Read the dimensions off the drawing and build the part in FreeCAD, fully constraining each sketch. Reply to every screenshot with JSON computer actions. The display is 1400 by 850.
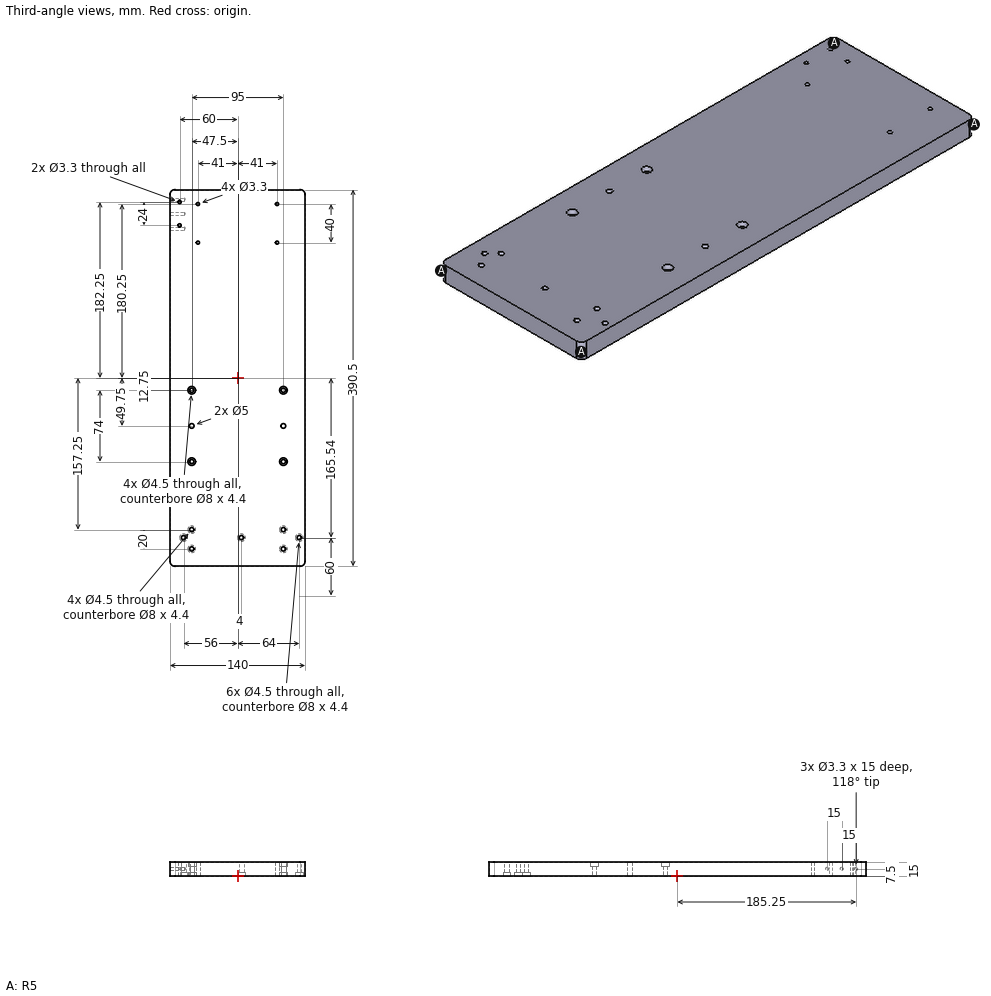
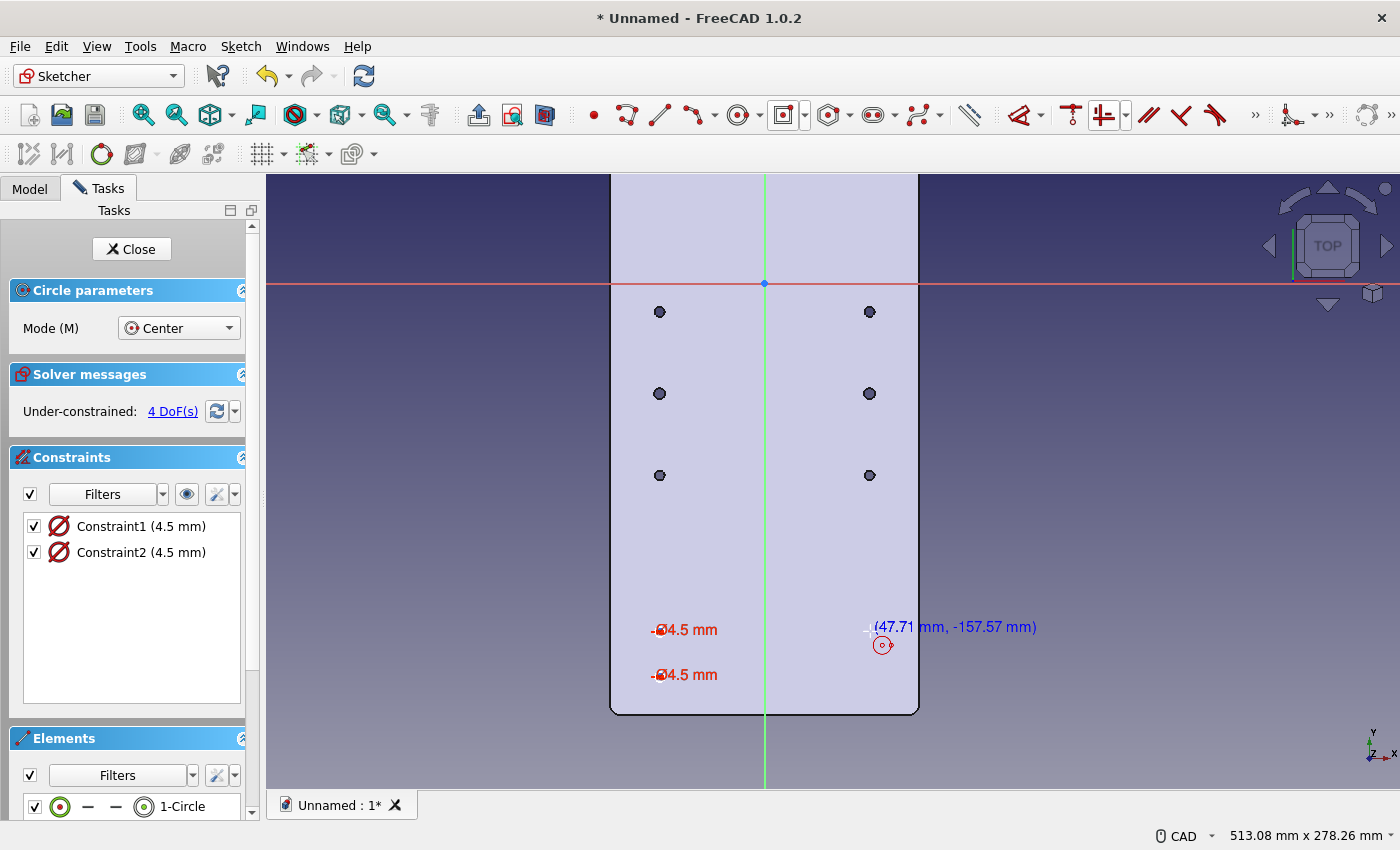
{"action": "left_click", "coordinate": [870, 631]}
{"action": "mouse_move", "coordinate": [873, 628]}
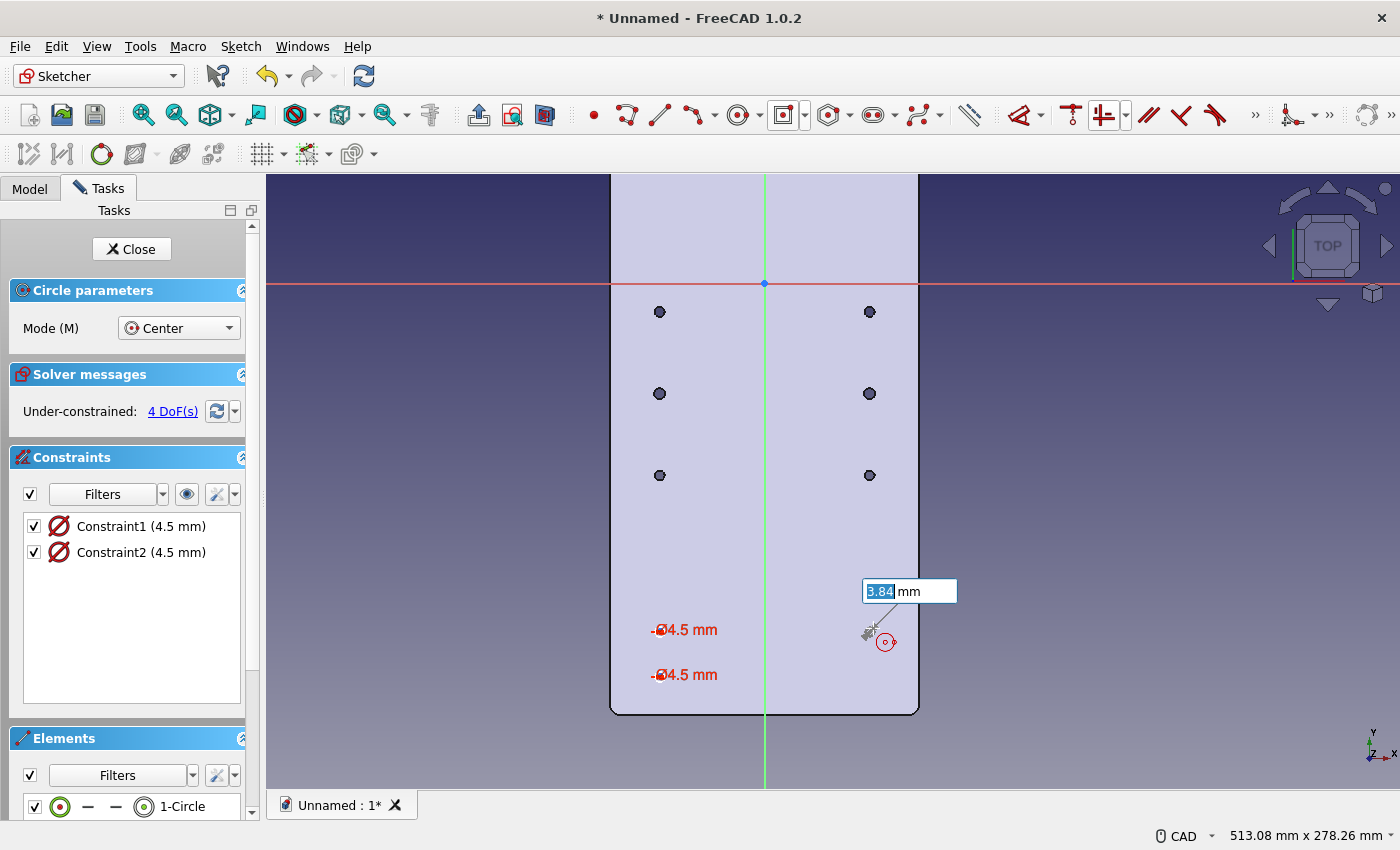
{"action": "type", "text": "4.5"}
{"action": "key", "text": "Return"}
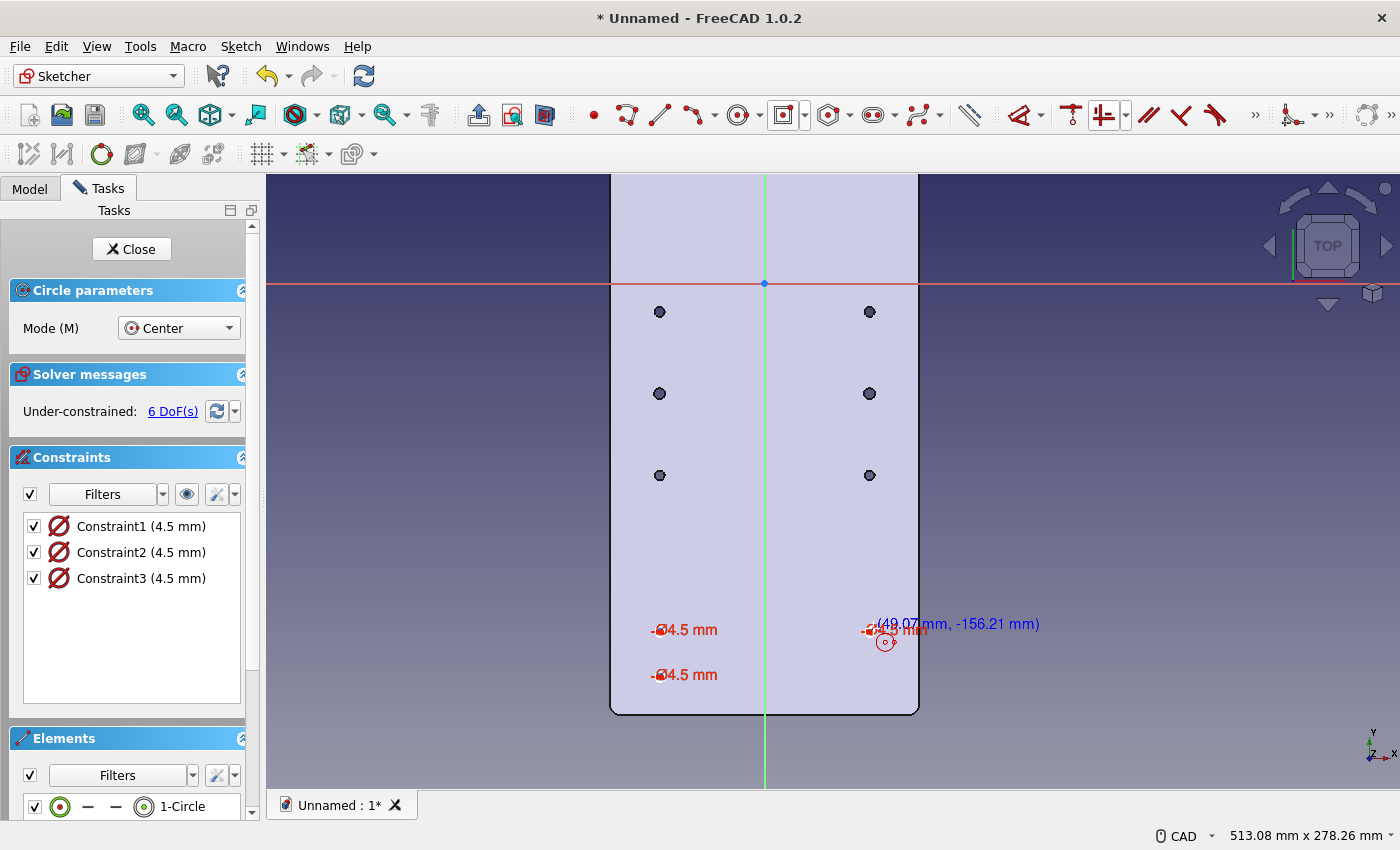
{"action": "scroll", "coordinate": [870, 676], "scroll_direction": "up", "scroll_amount": 8}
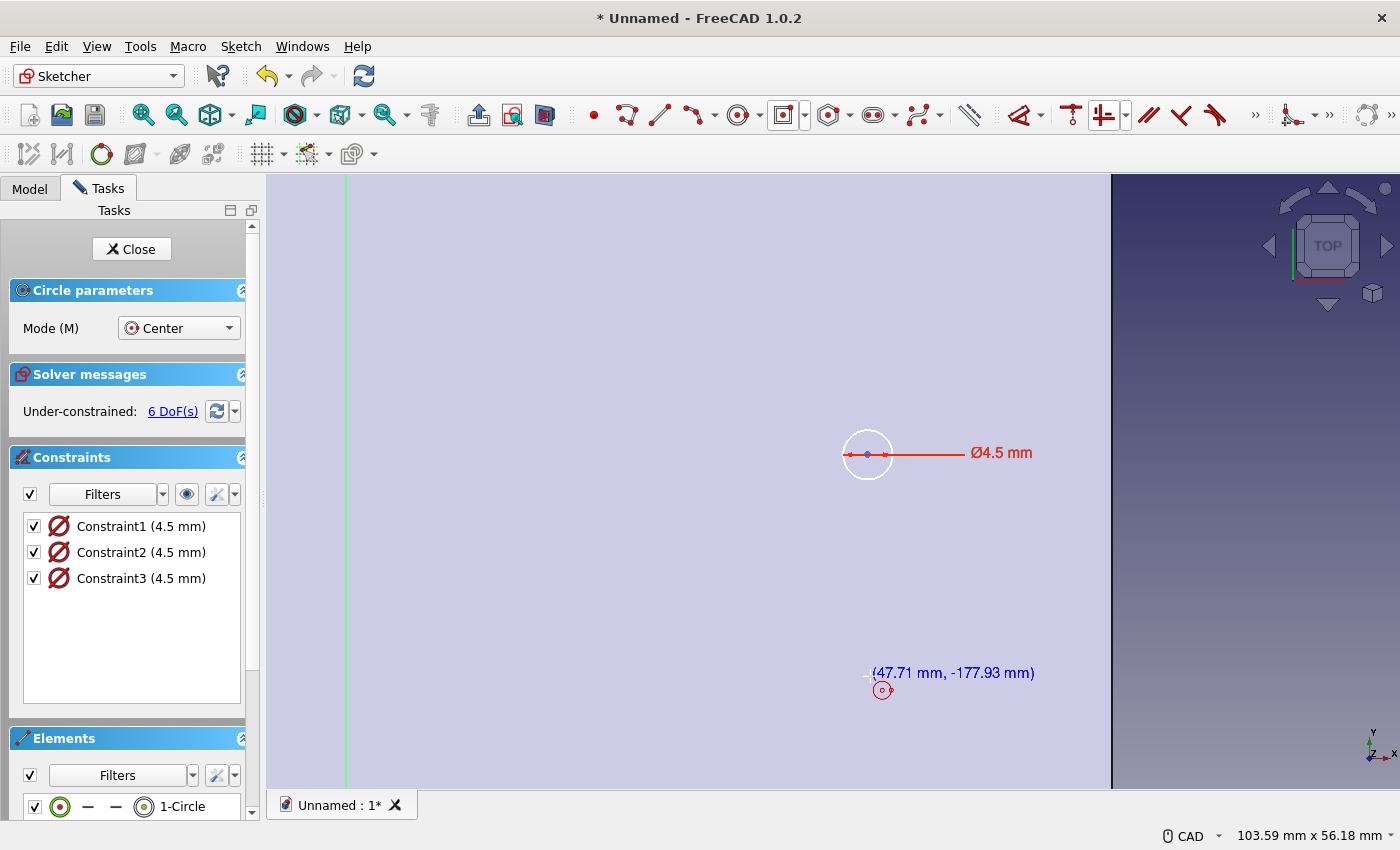
{"action": "scroll", "coordinate": [870, 676], "scroll_direction": "down", "scroll_amount": 8}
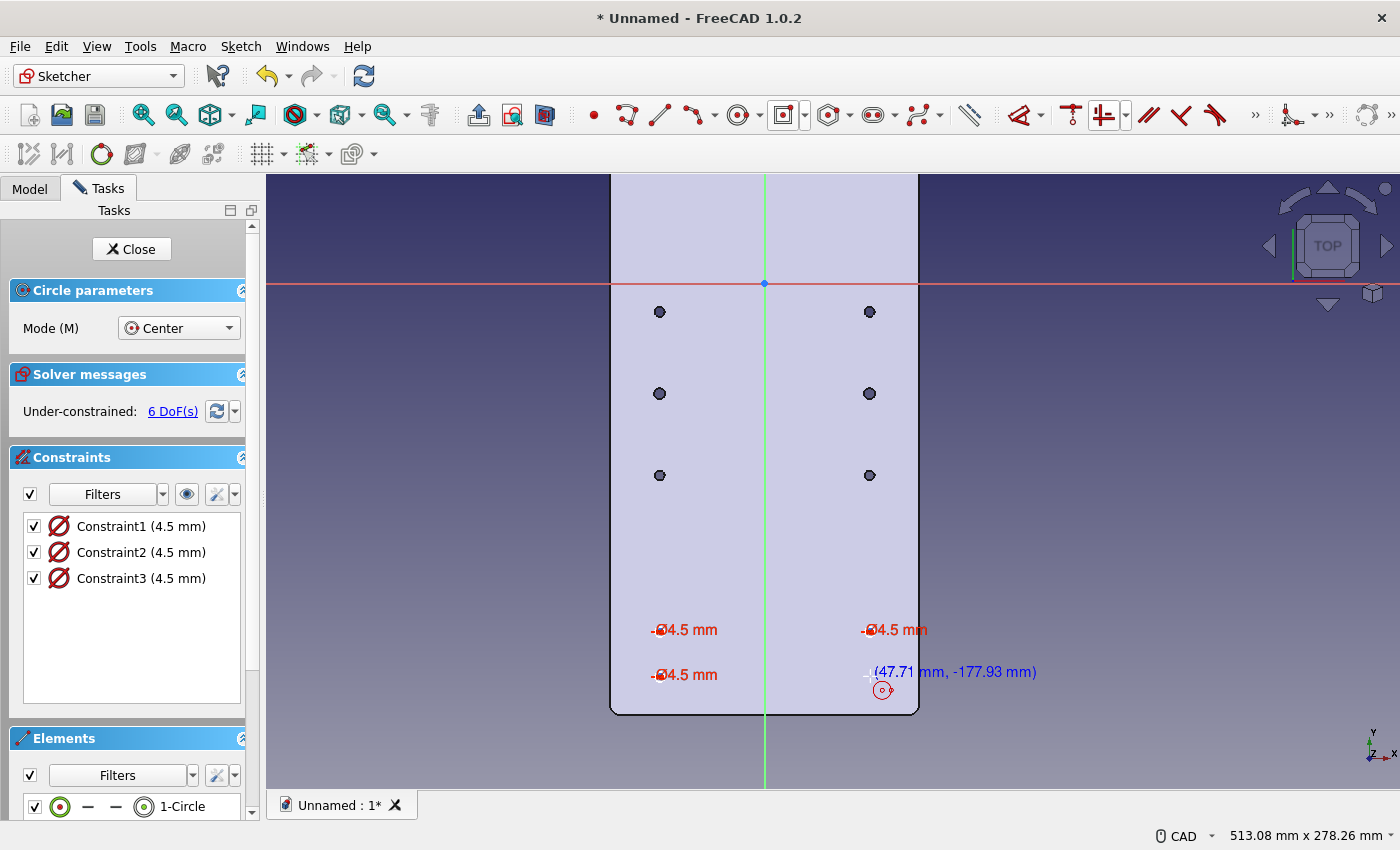
{"action": "left_click", "coordinate": [870, 676]}
{"action": "mouse_move", "coordinate": [873, 672]}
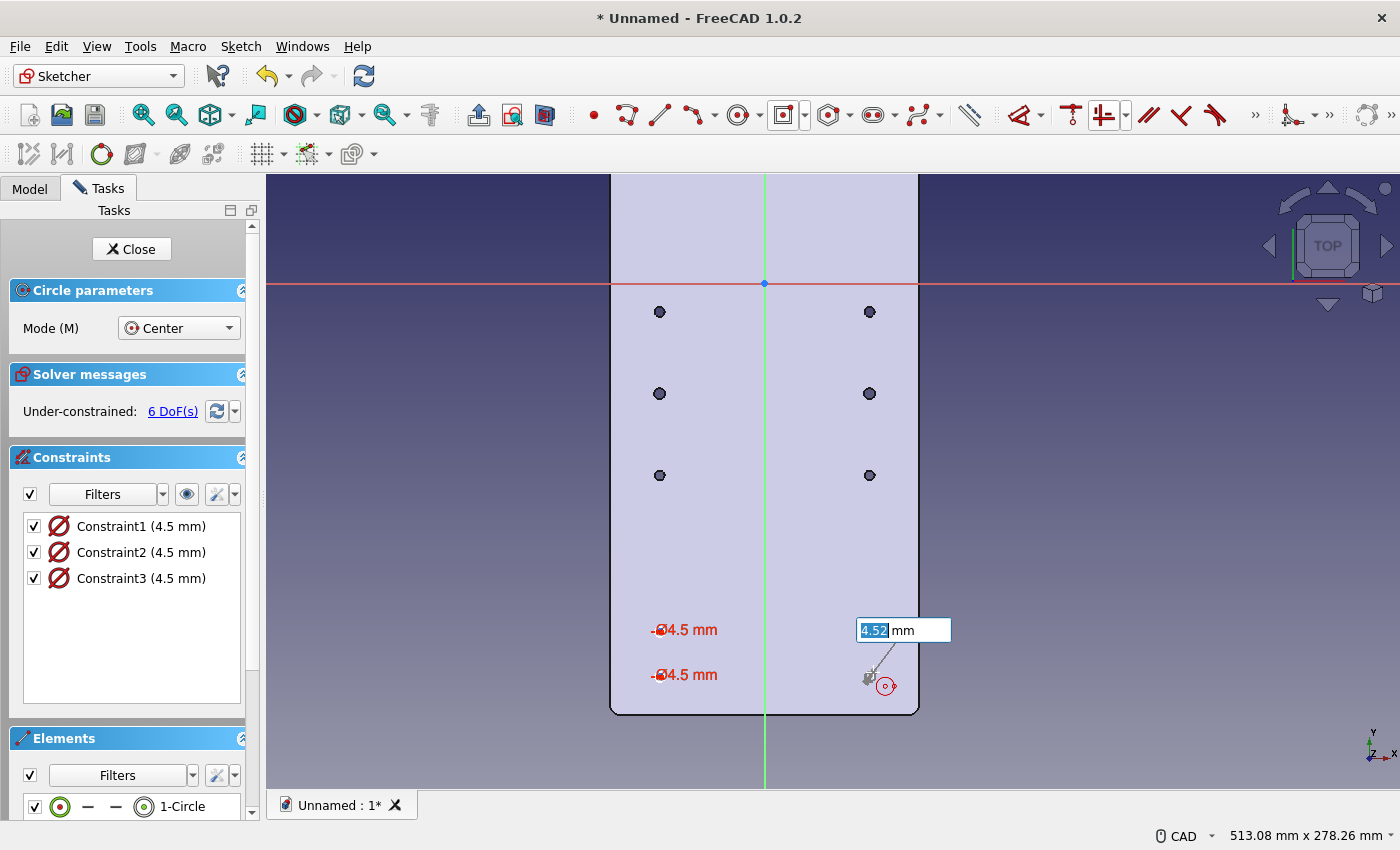
{"action": "type", "text": "4.5"}
{"action": "key", "text": "Return"}
{"action": "key", "text": "Escape"}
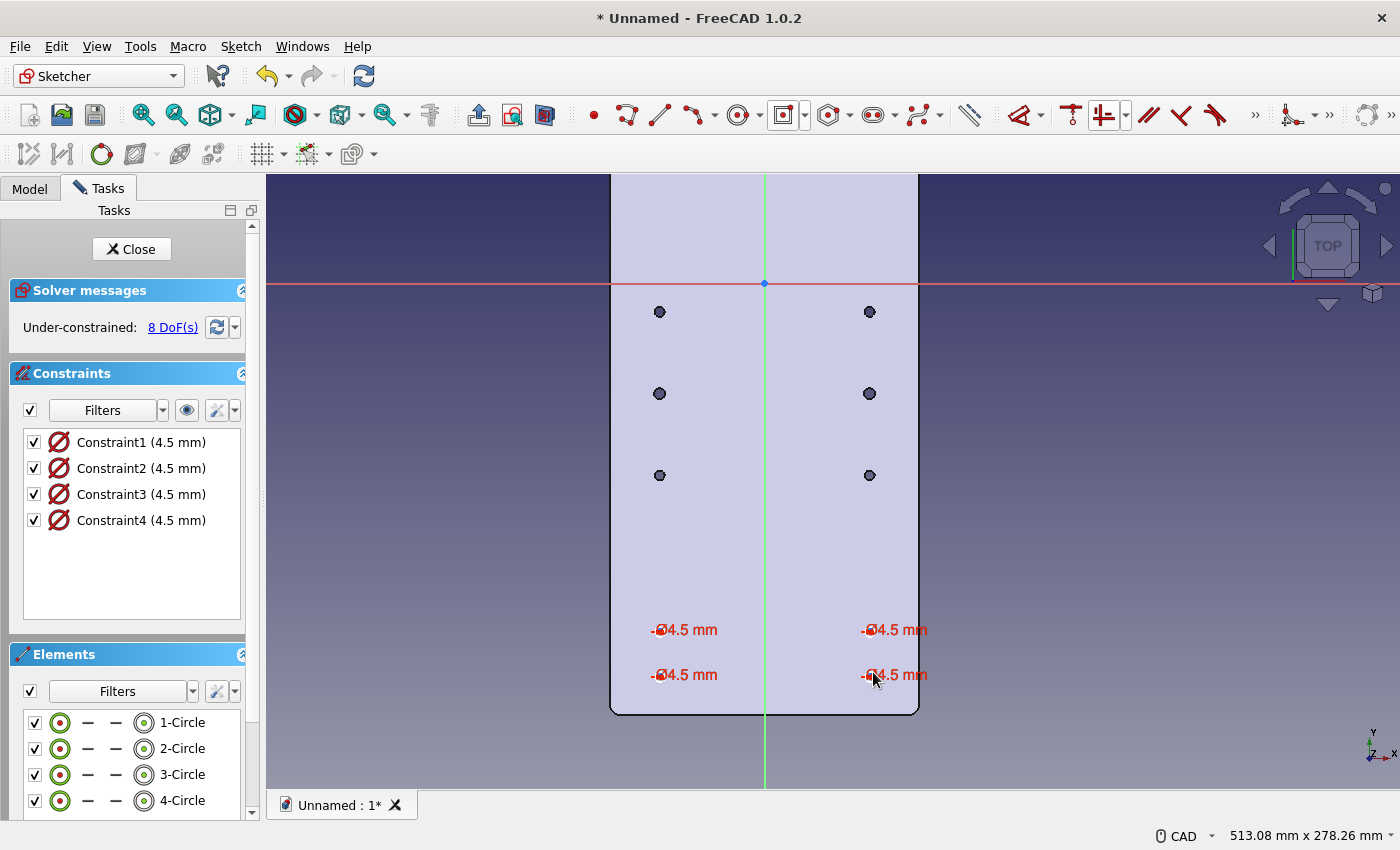
{"action": "left_click", "coordinate": [660, 632]}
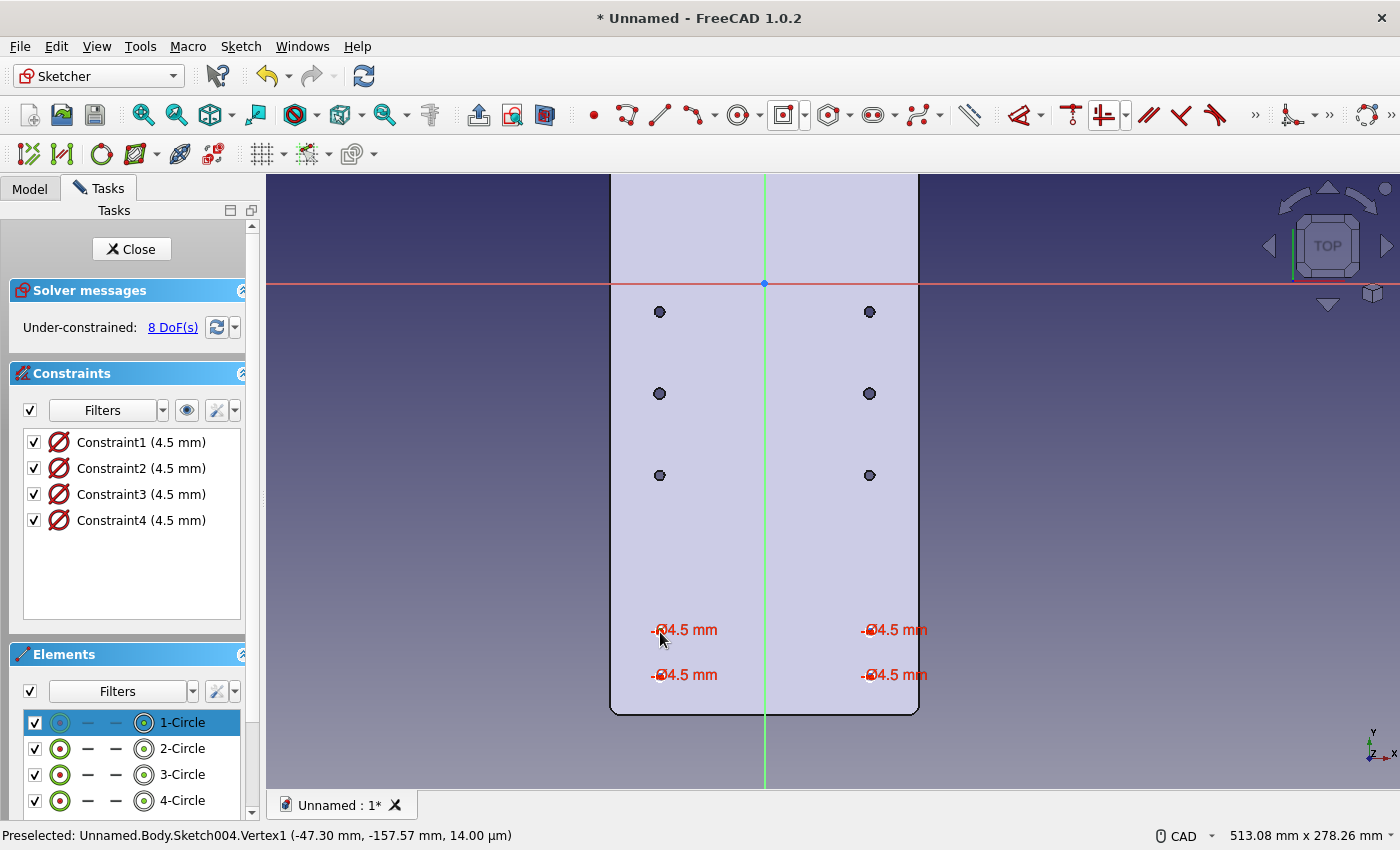
{"action": "left_click", "coordinate": [660, 677]}